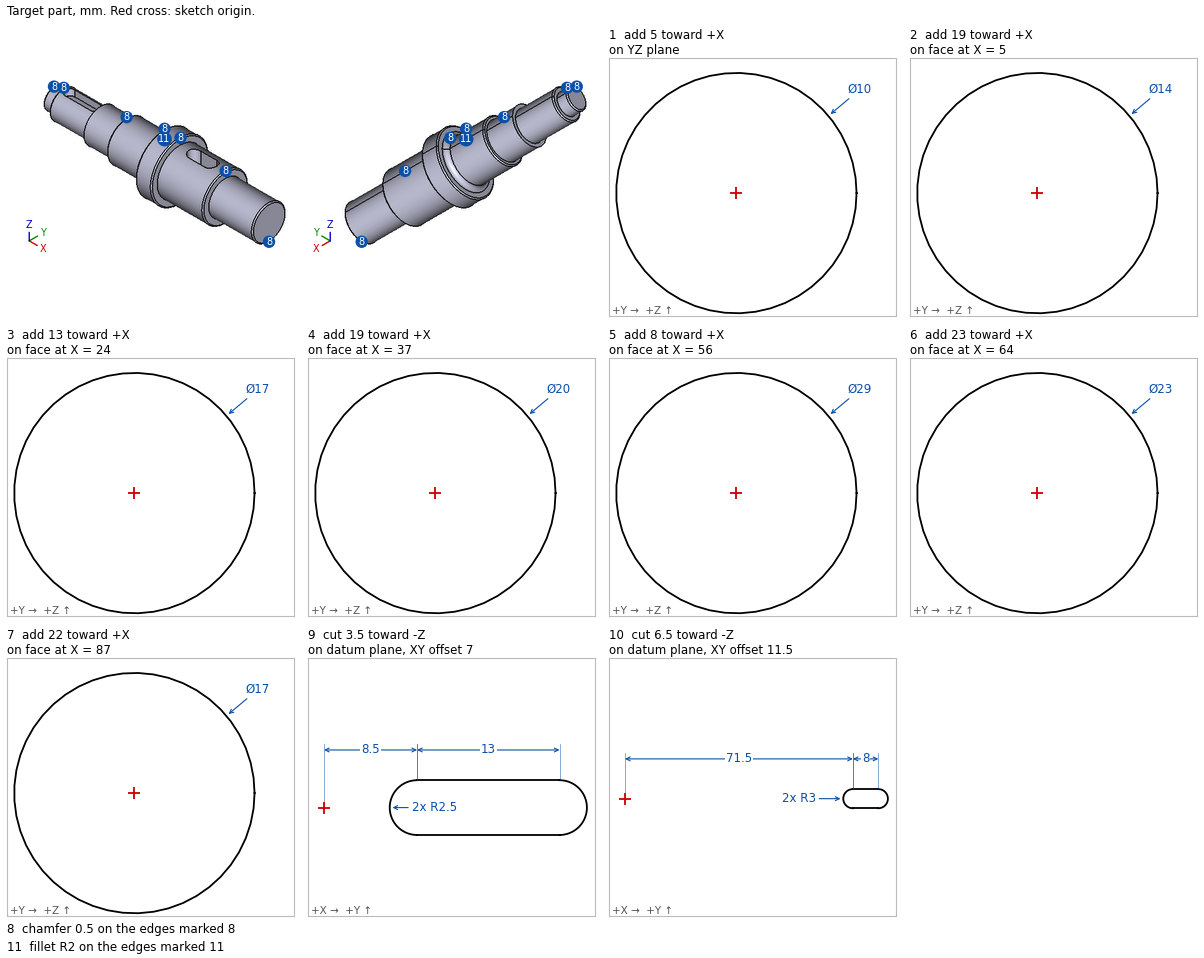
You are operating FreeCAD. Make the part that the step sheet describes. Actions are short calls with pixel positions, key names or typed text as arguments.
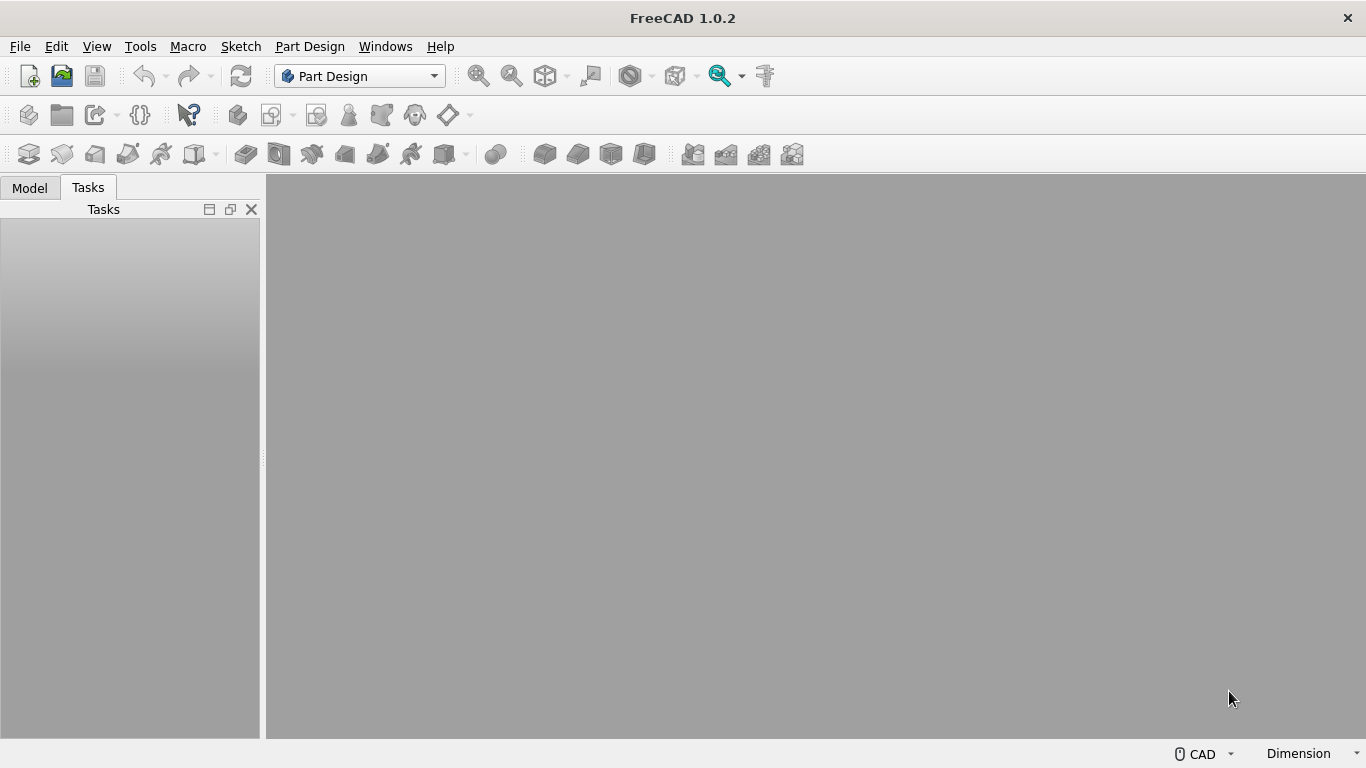
click(29, 76)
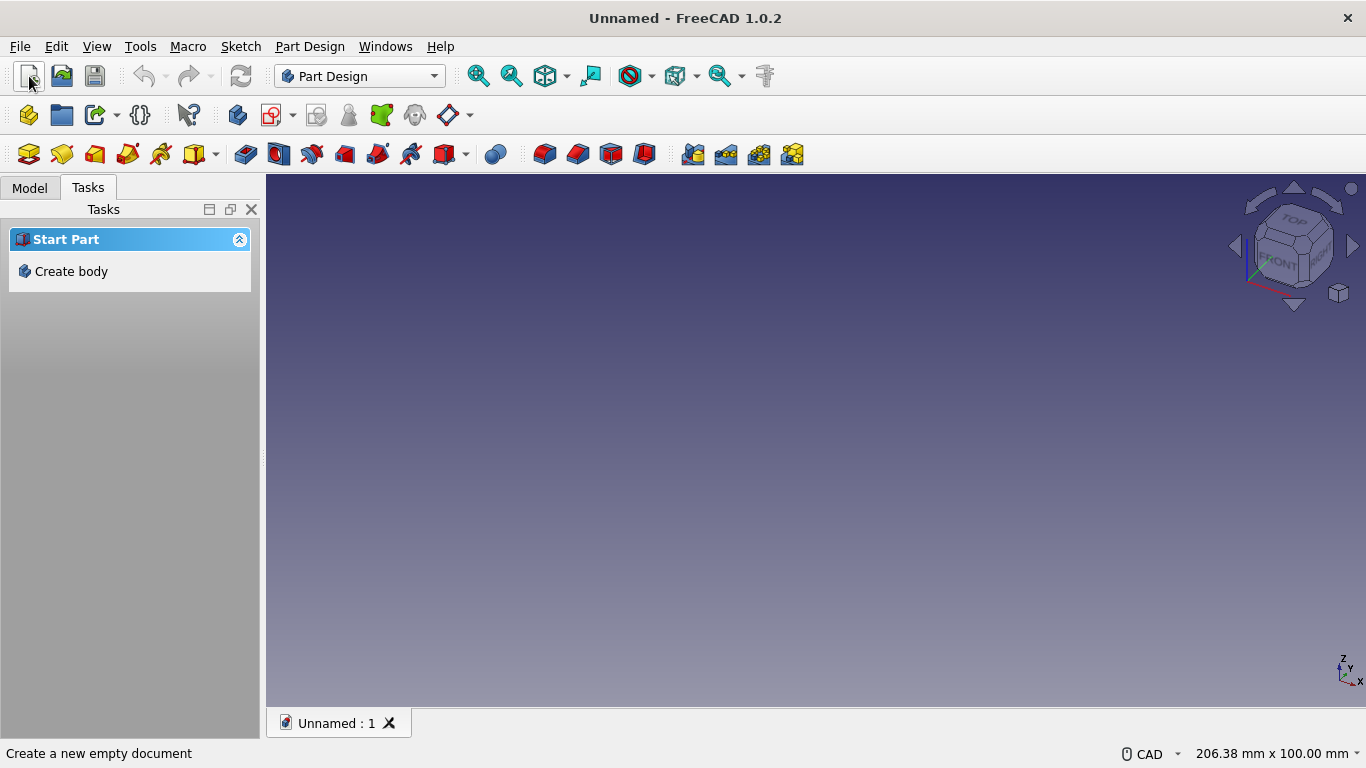
click(270, 116)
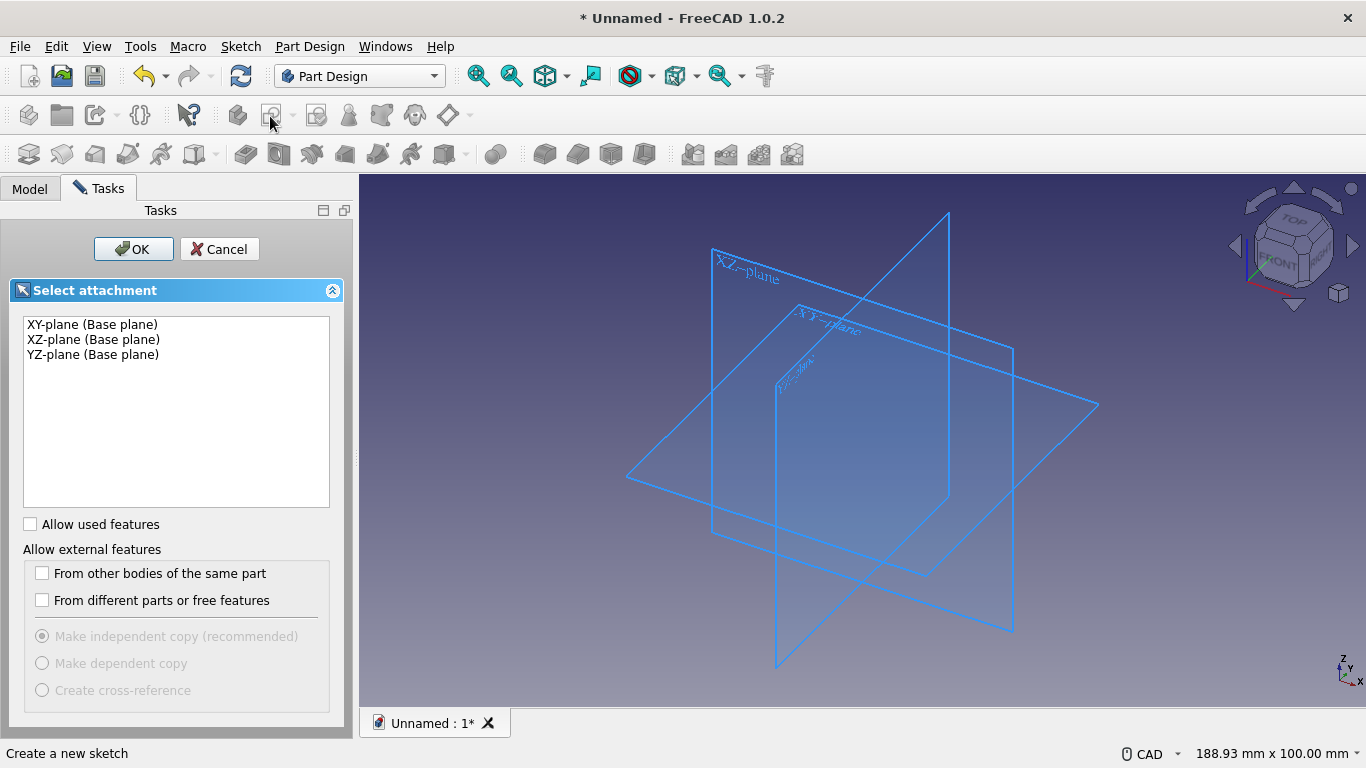
click(84, 354)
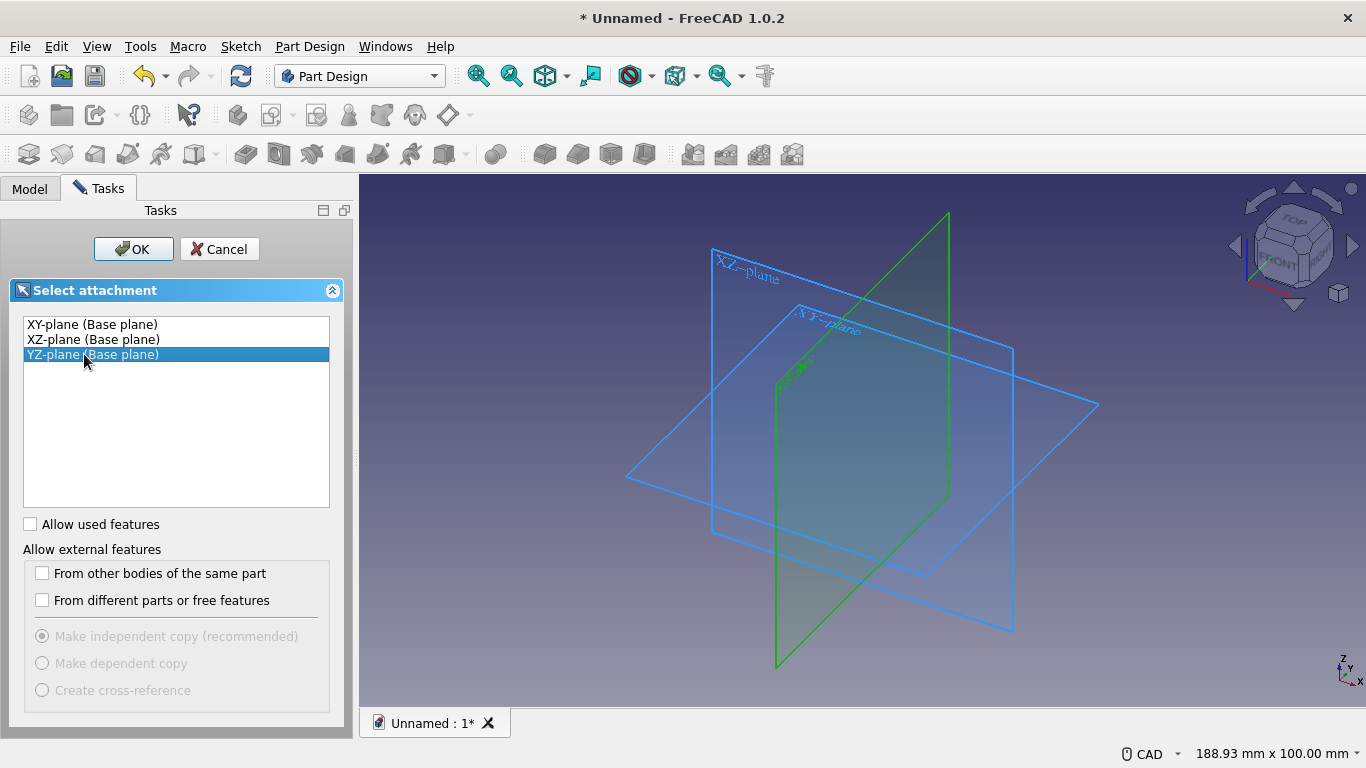
click(134, 249)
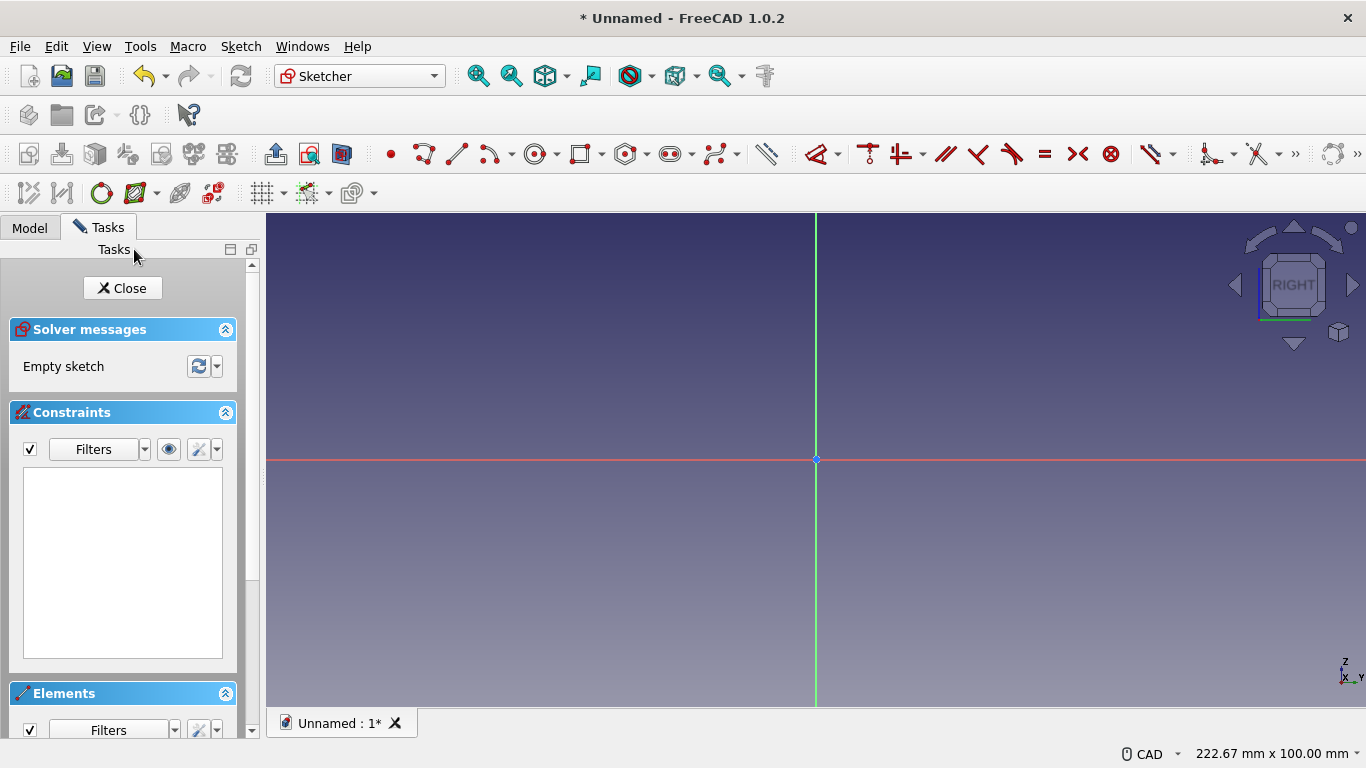
scroll(830, 460, up, 9)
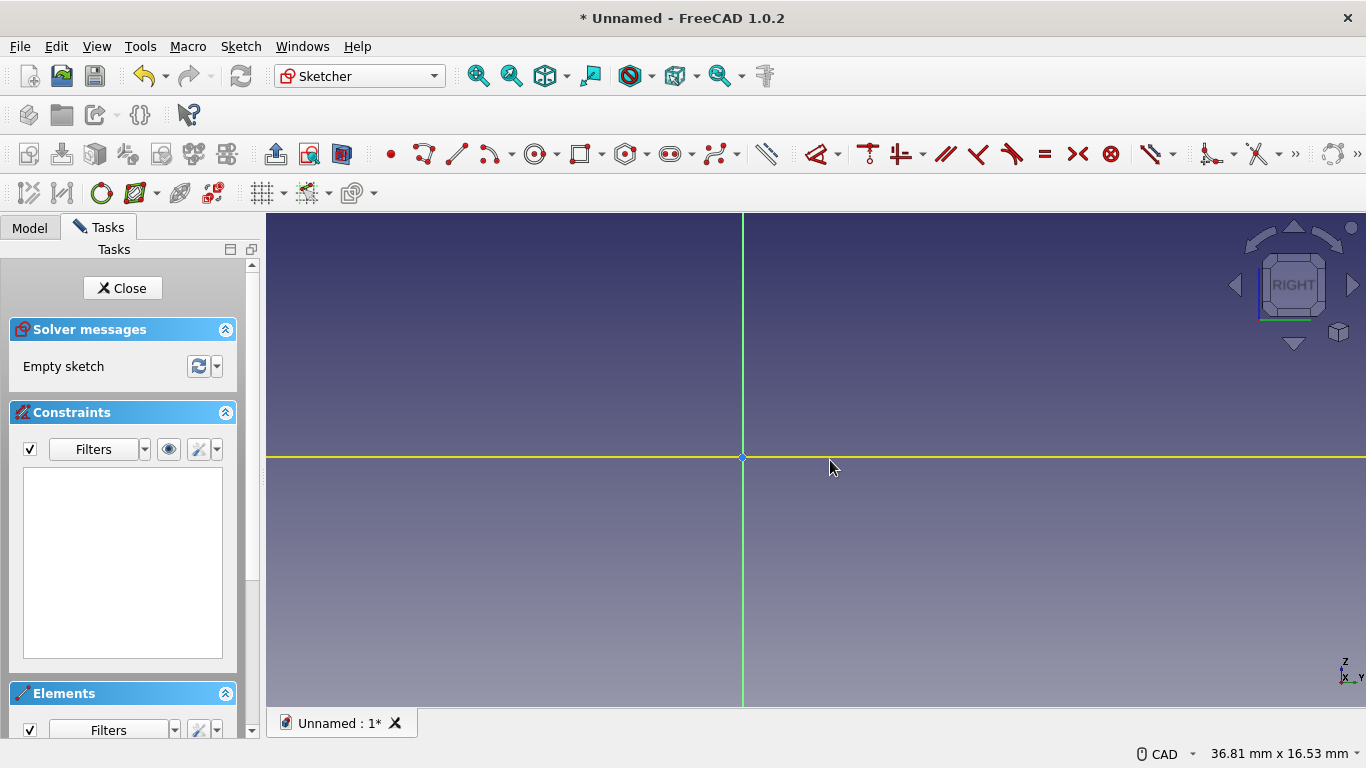
click(534, 154)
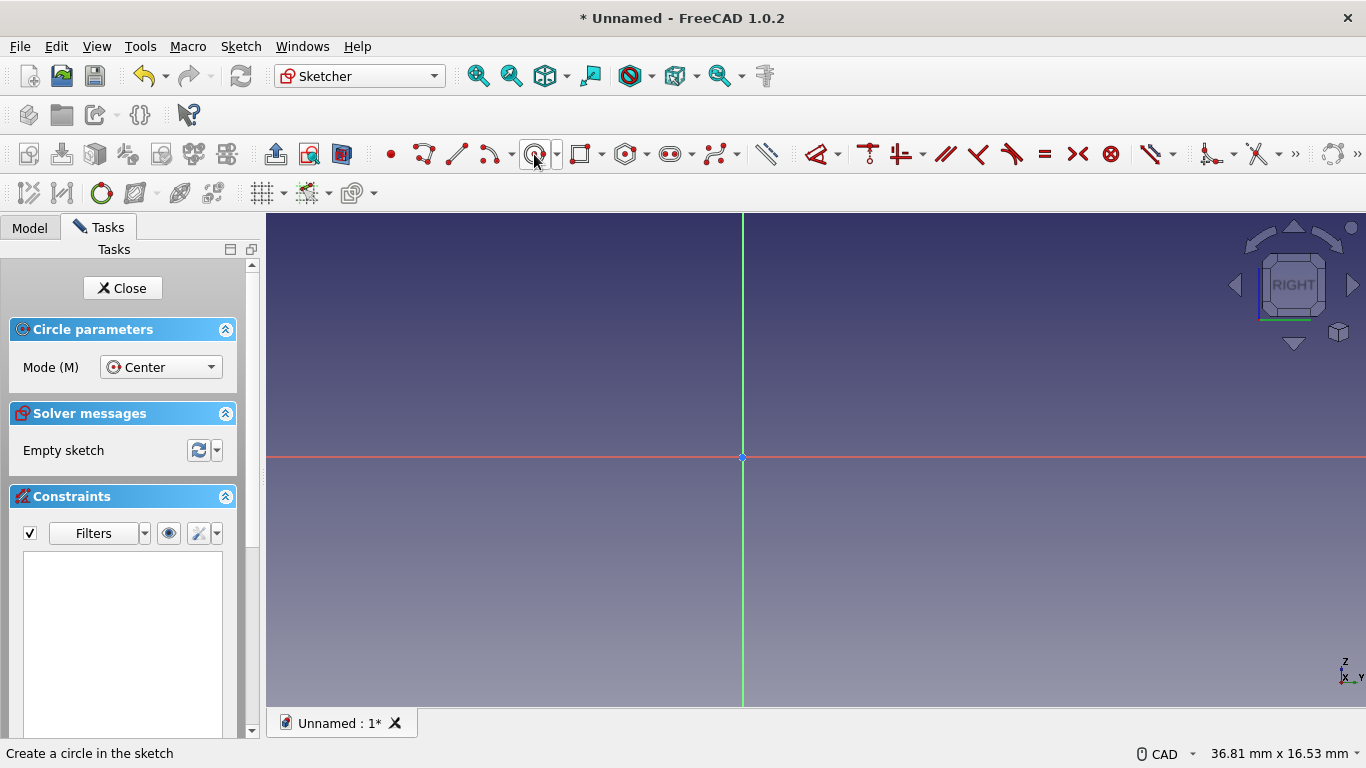
click(743, 457)
move(848, 352)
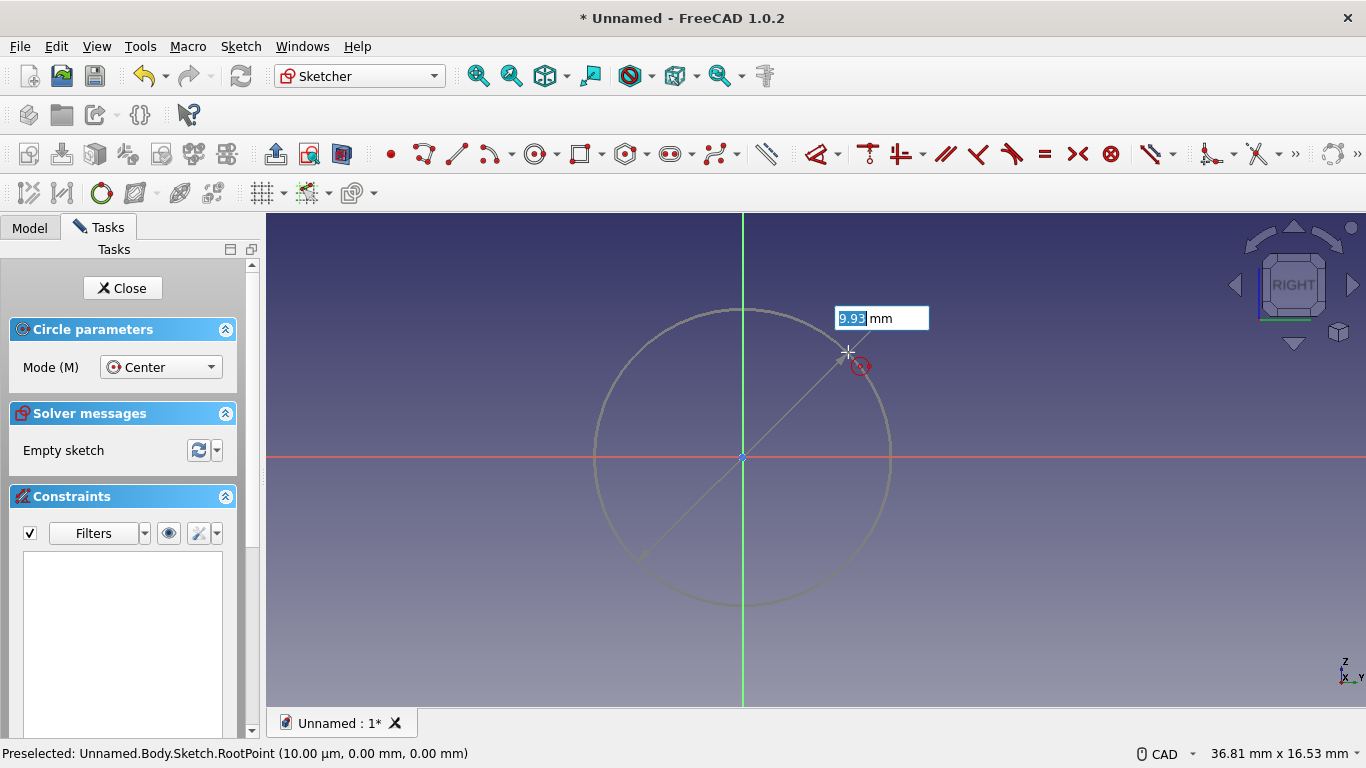
text(10)
key(Return)
key(Escape)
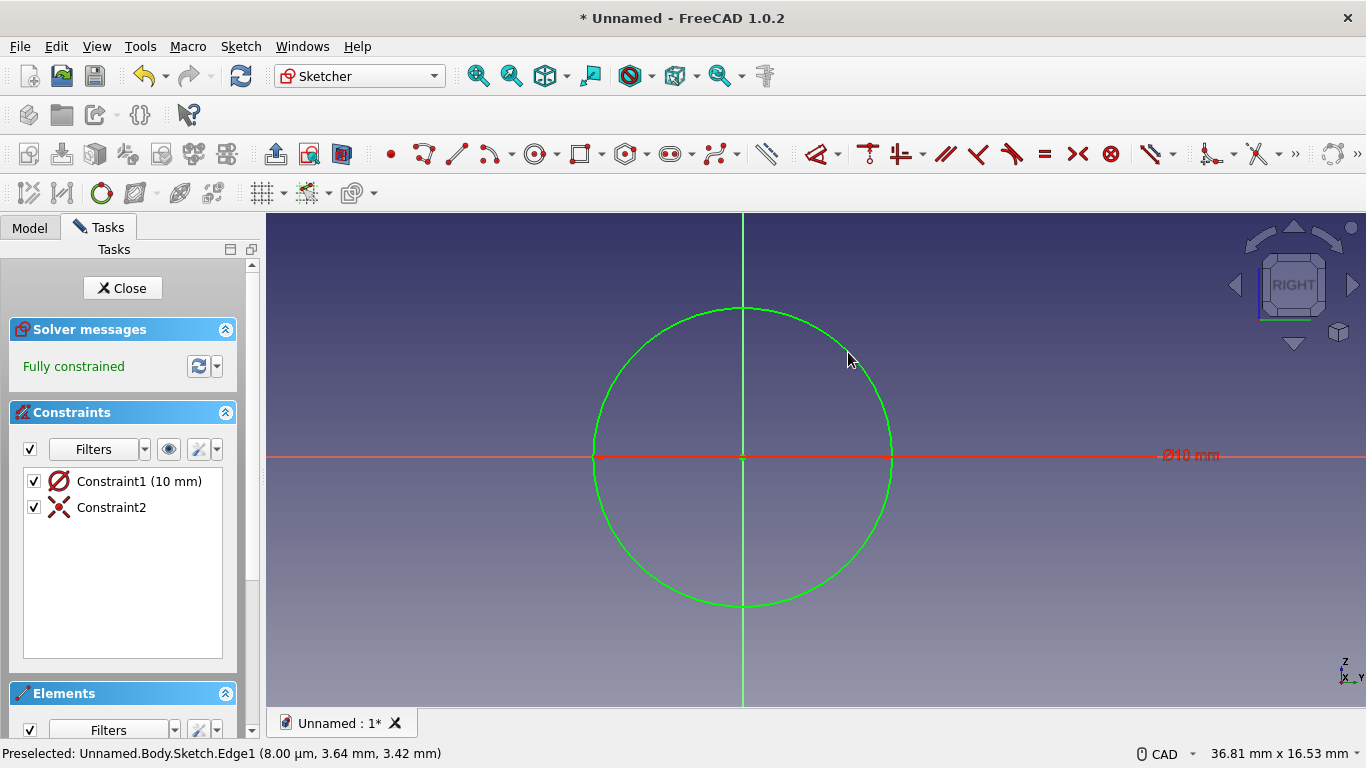
click(123, 288)